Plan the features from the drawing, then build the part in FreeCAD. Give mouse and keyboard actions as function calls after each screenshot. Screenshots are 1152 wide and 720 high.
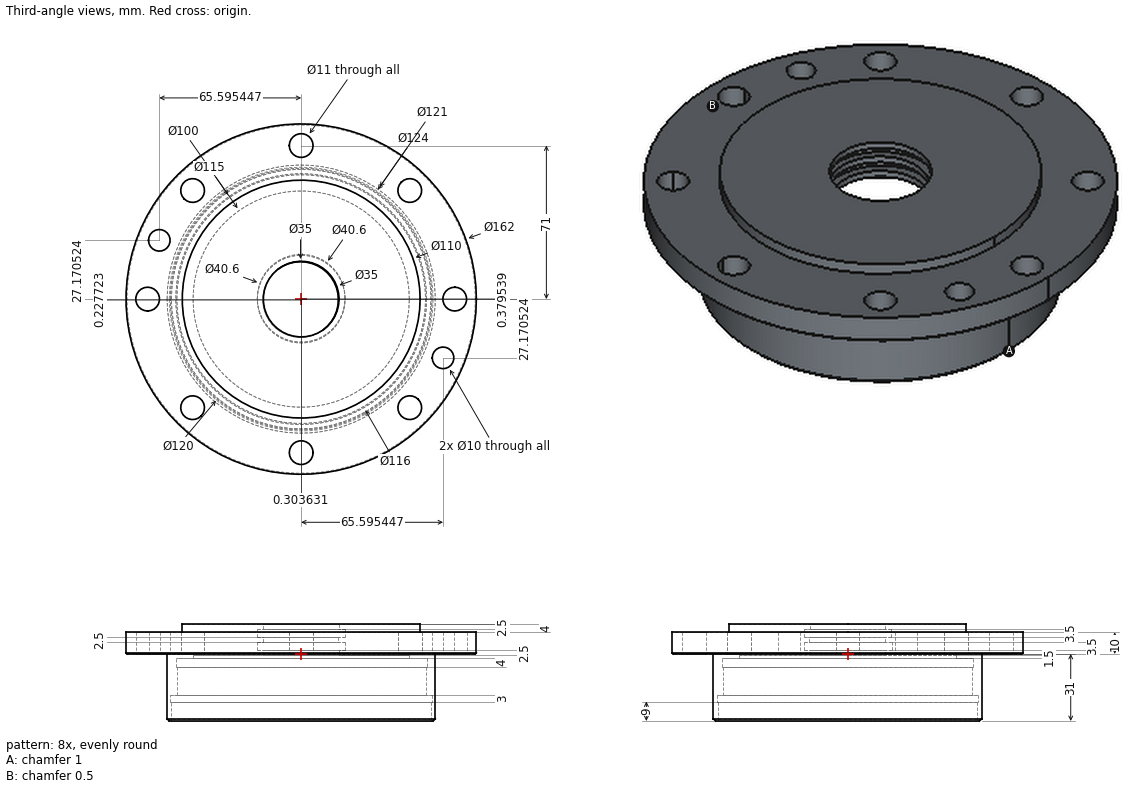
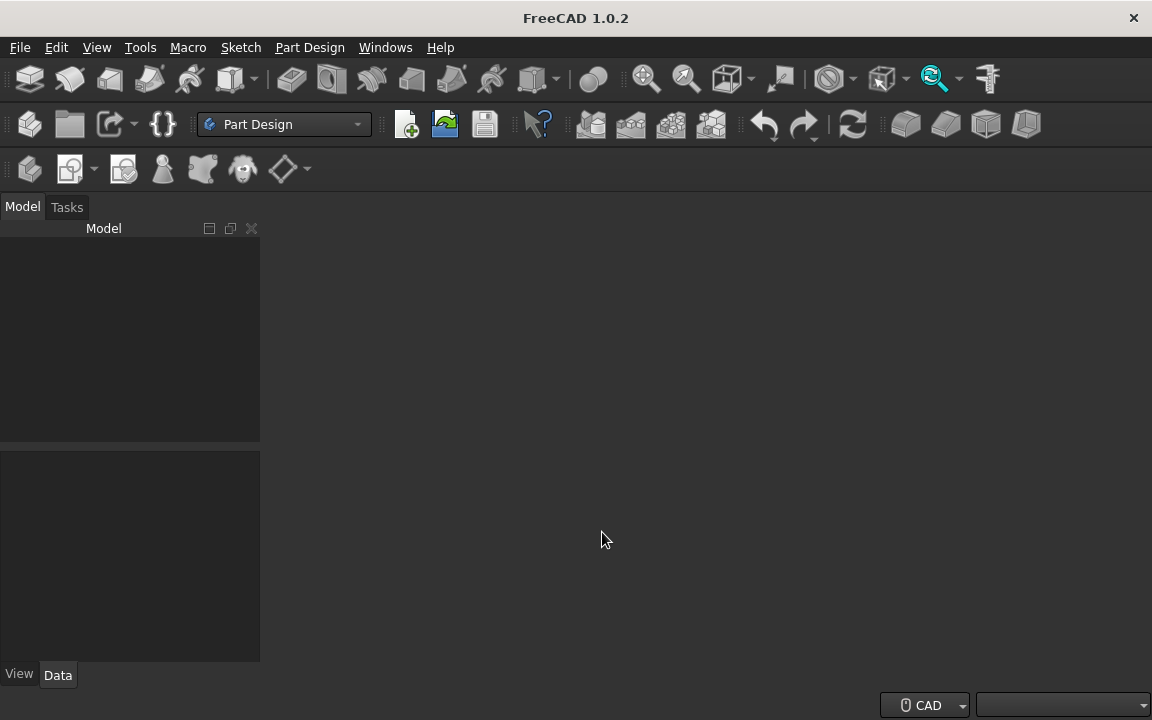
click(406, 124)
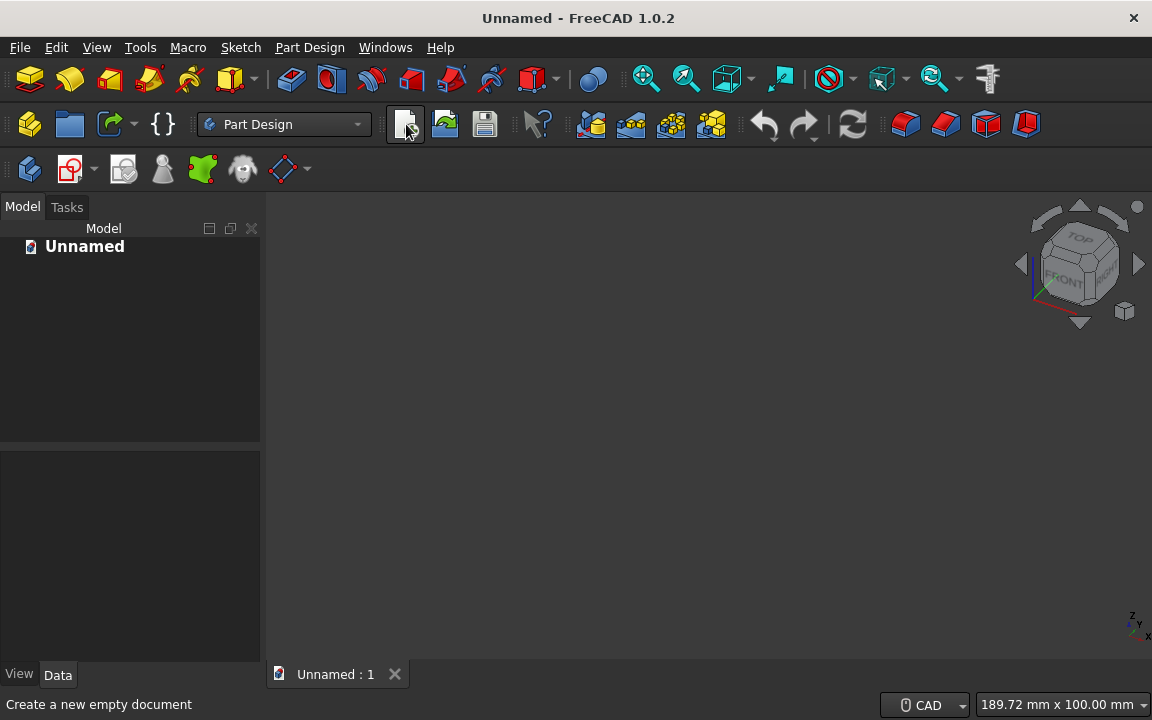
click(70, 170)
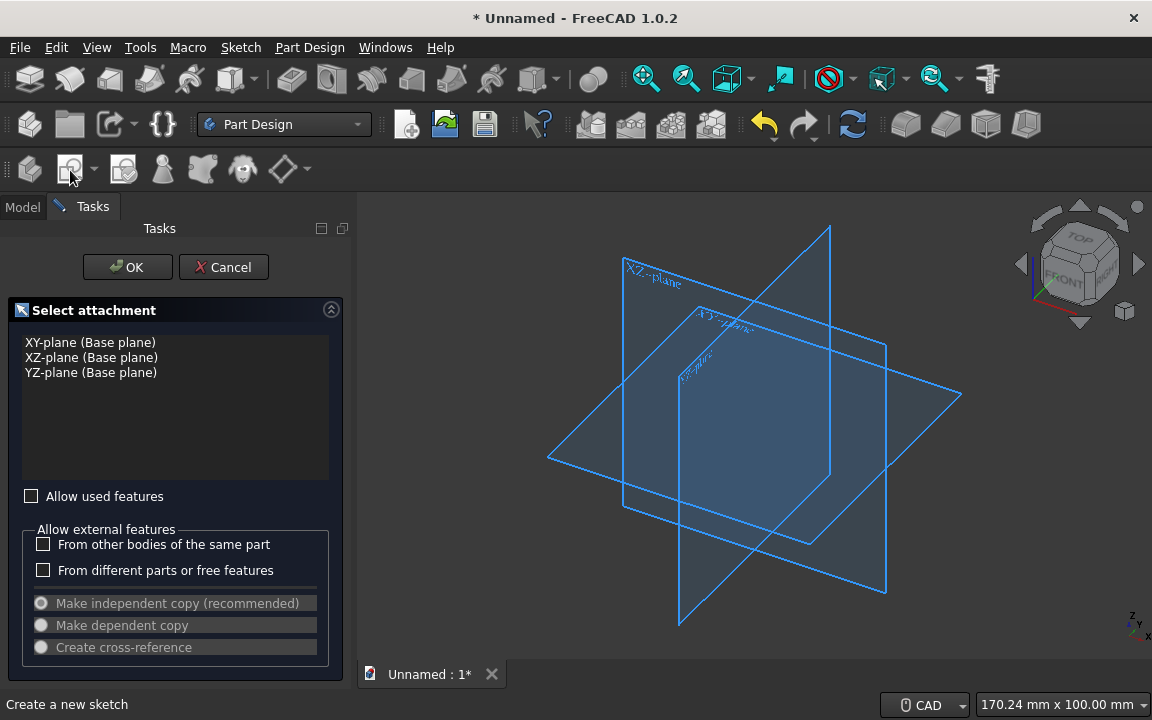
click(82, 342)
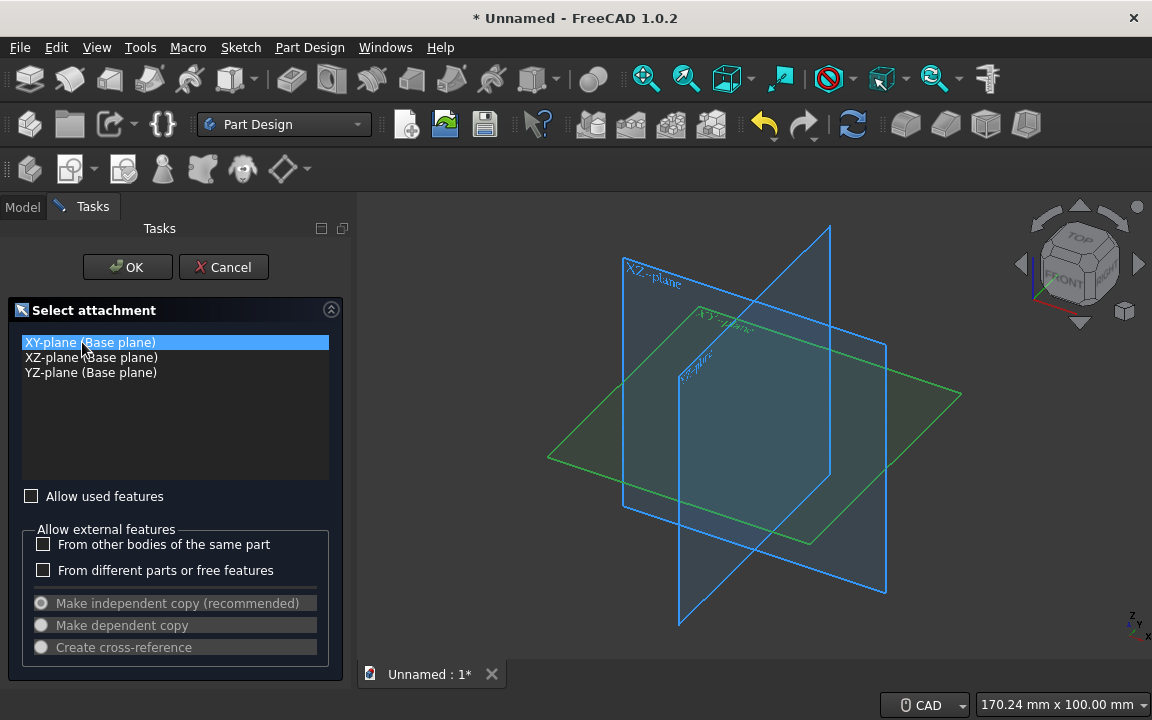
click(128, 267)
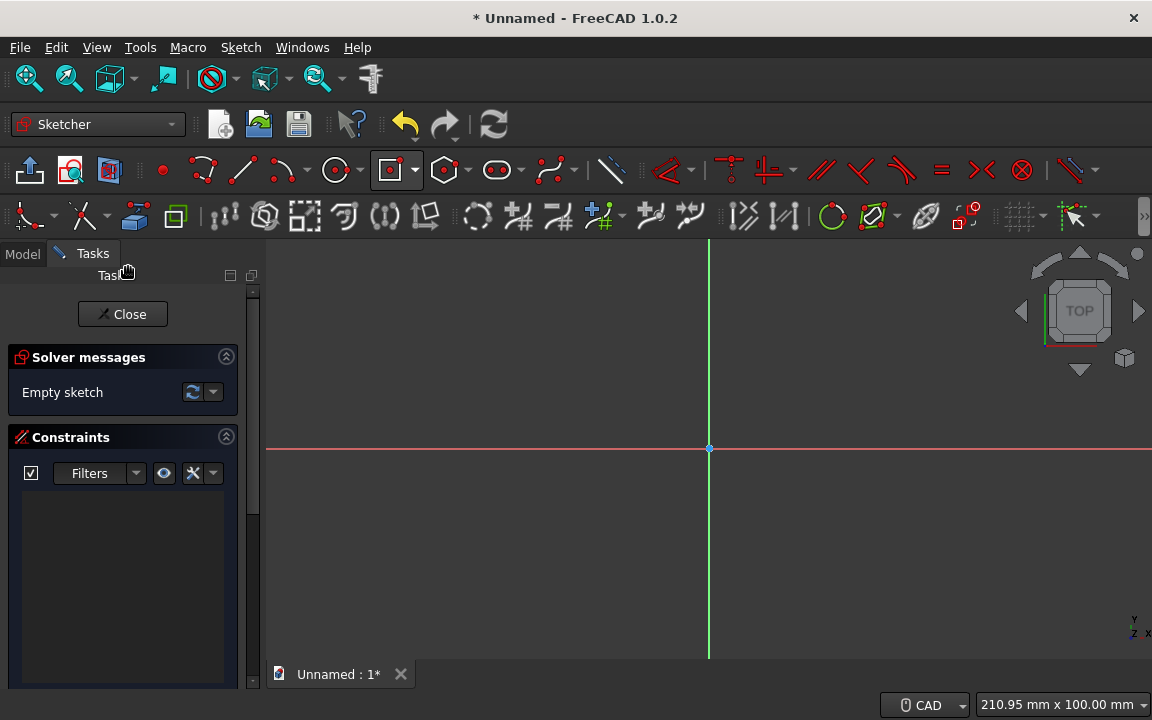
scroll(601, 449, down, 5)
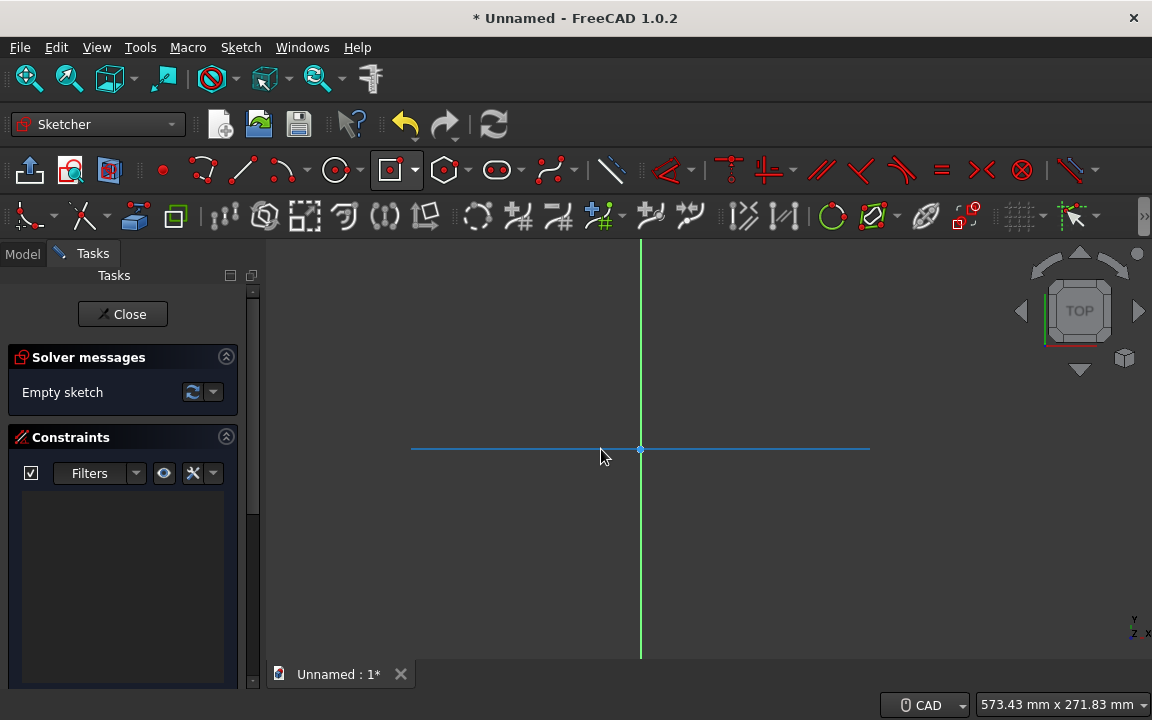
click(336, 170)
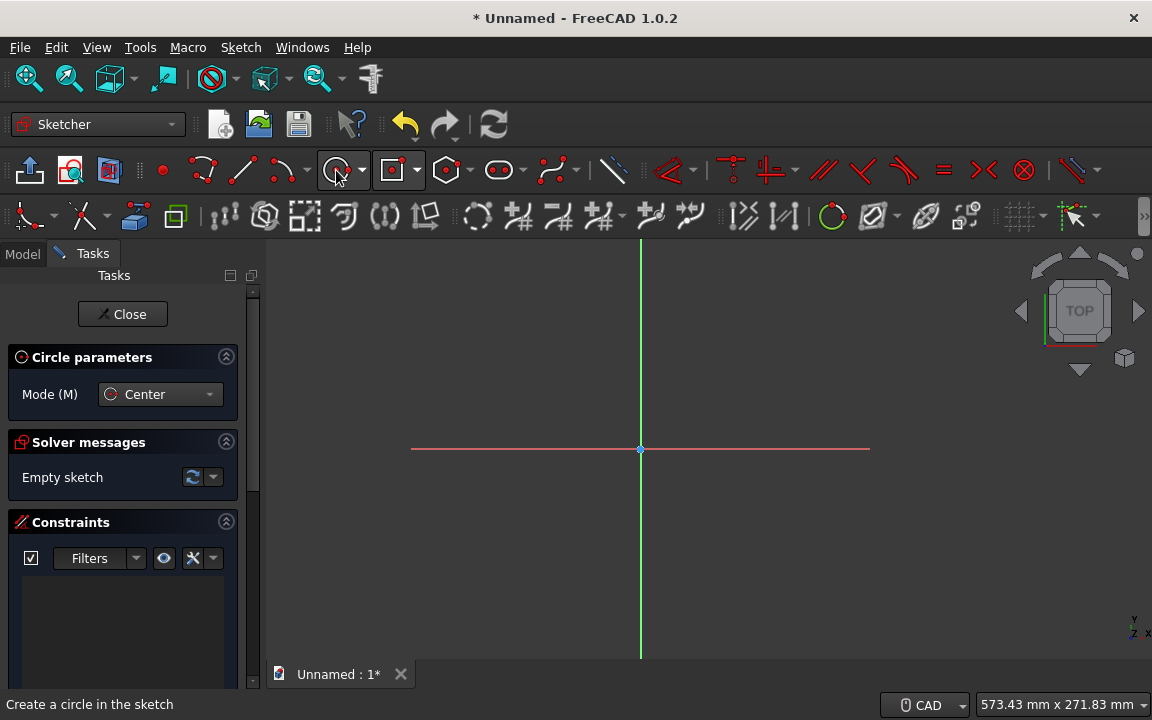
click(641, 449)
click(729, 361)
key(Escape)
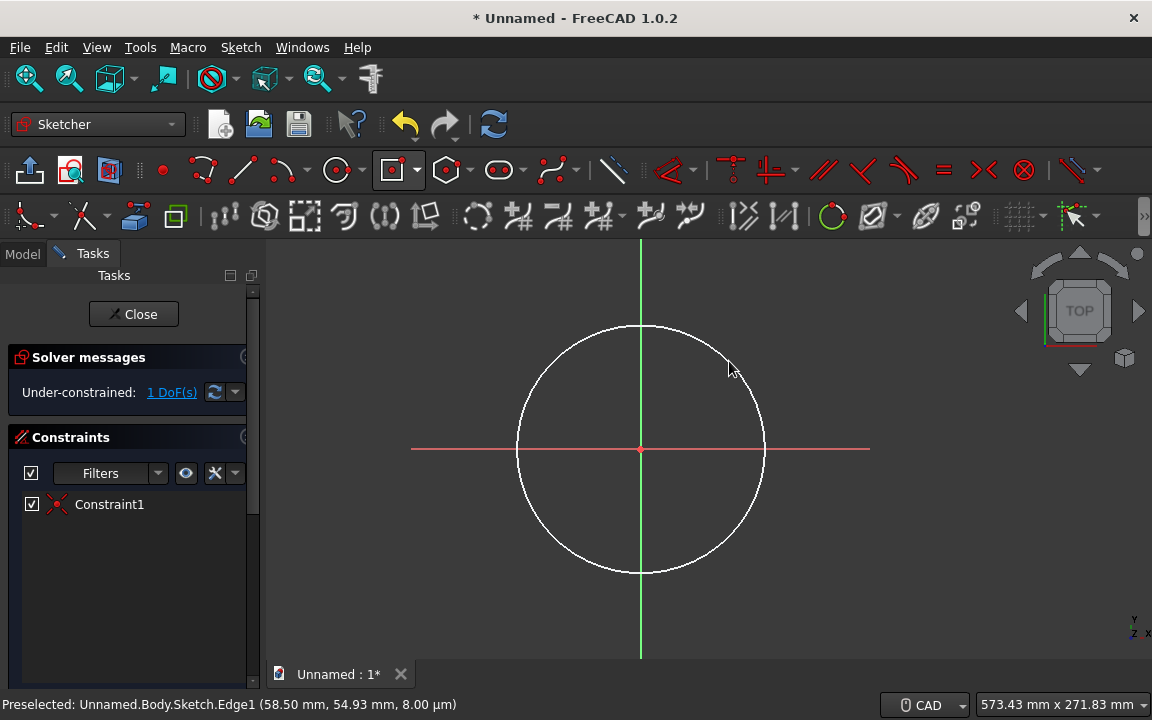
click(668, 170)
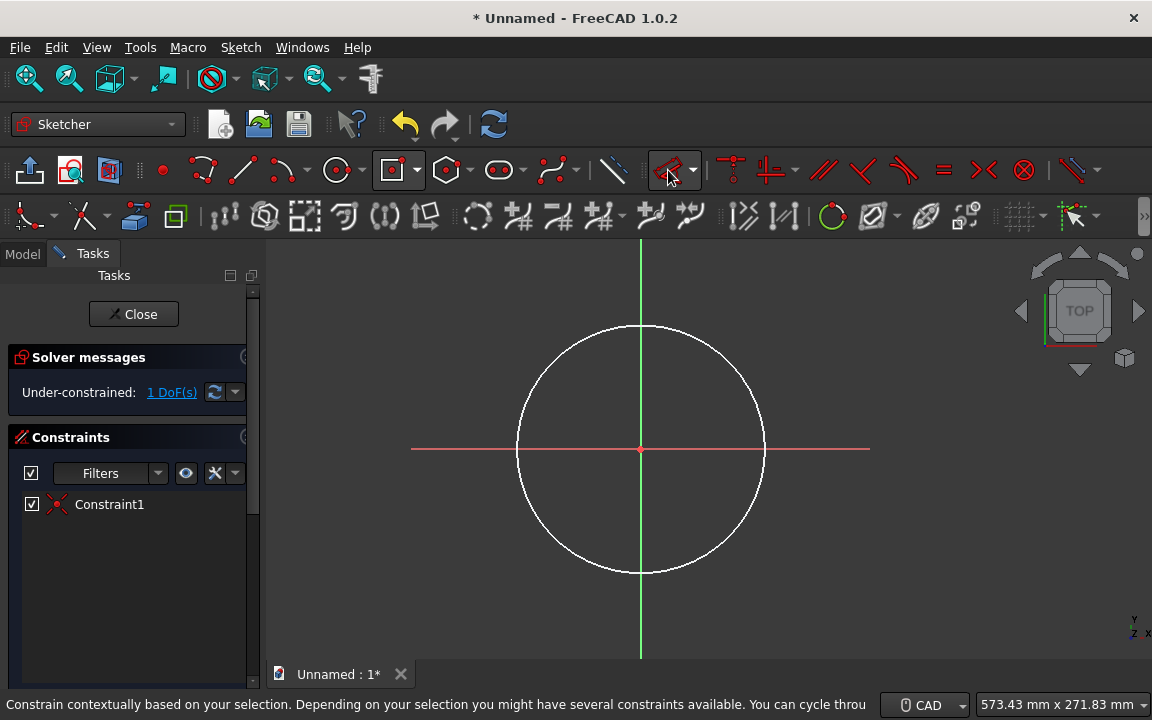
click(728, 361)
click(750, 338)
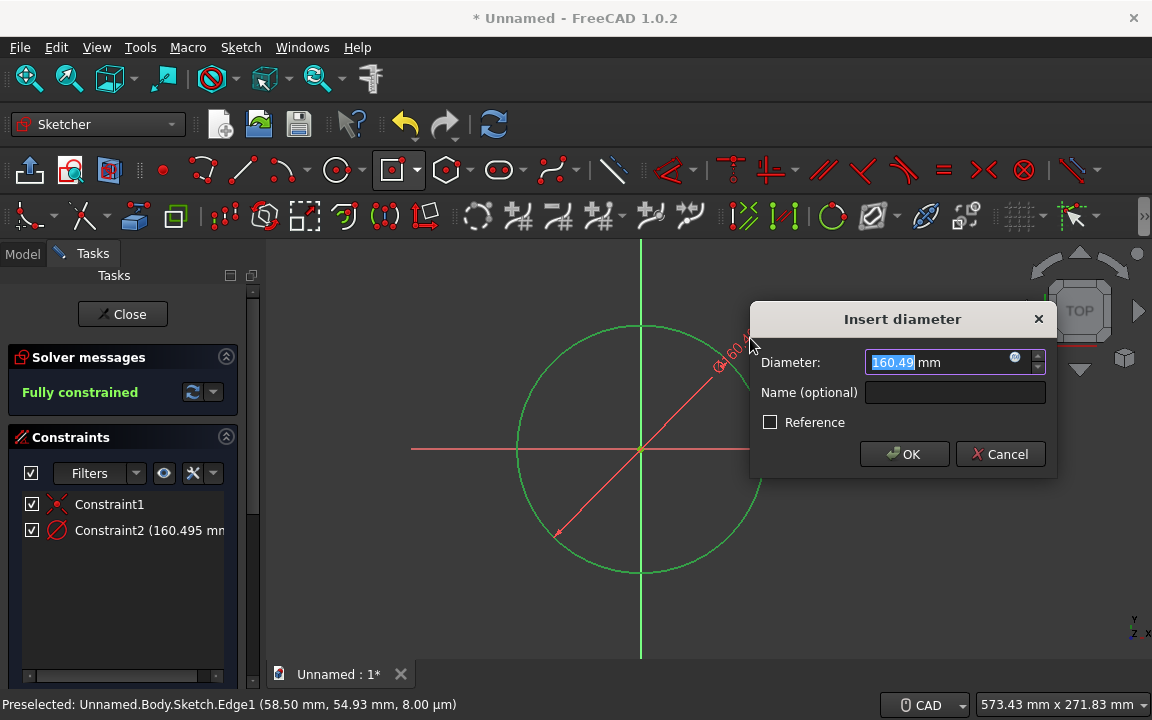
text(162)
key(Return)
key(Escape)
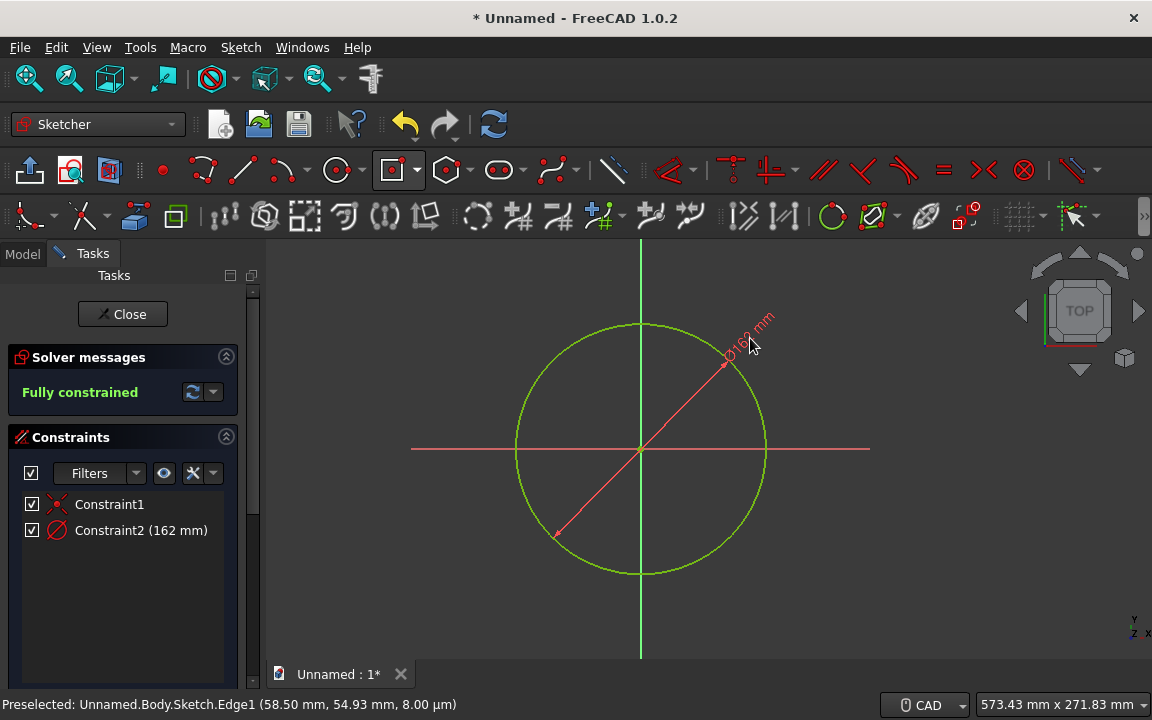
click(123, 314)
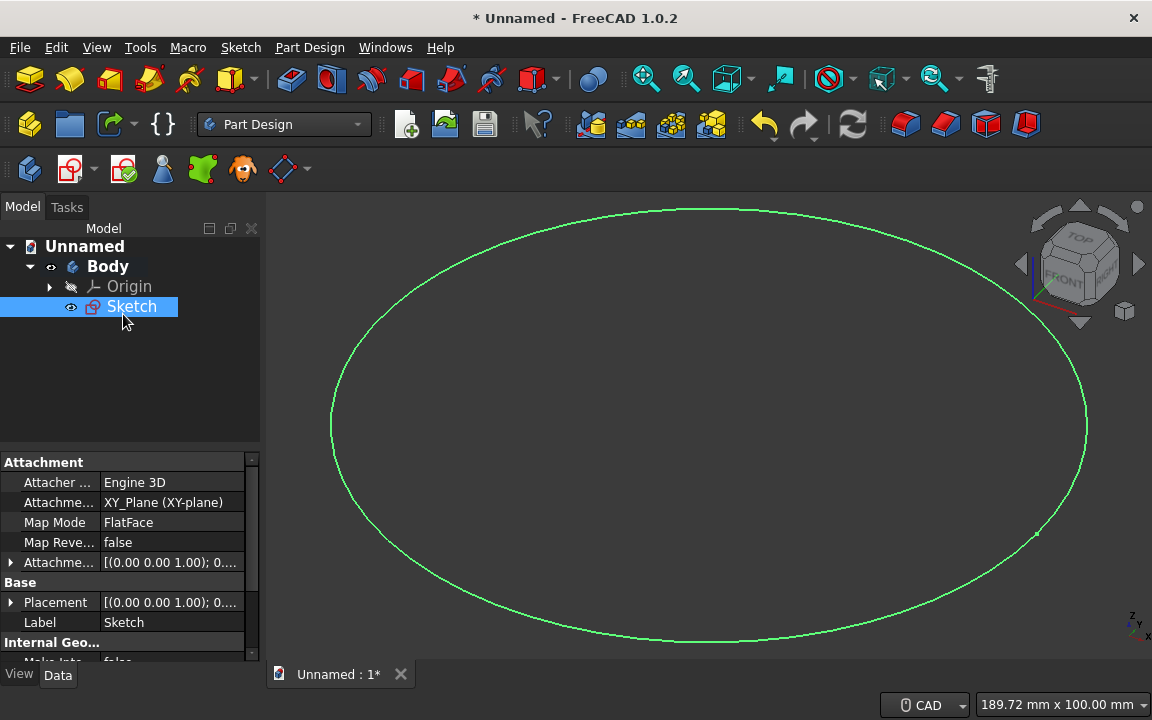
click(30, 80)